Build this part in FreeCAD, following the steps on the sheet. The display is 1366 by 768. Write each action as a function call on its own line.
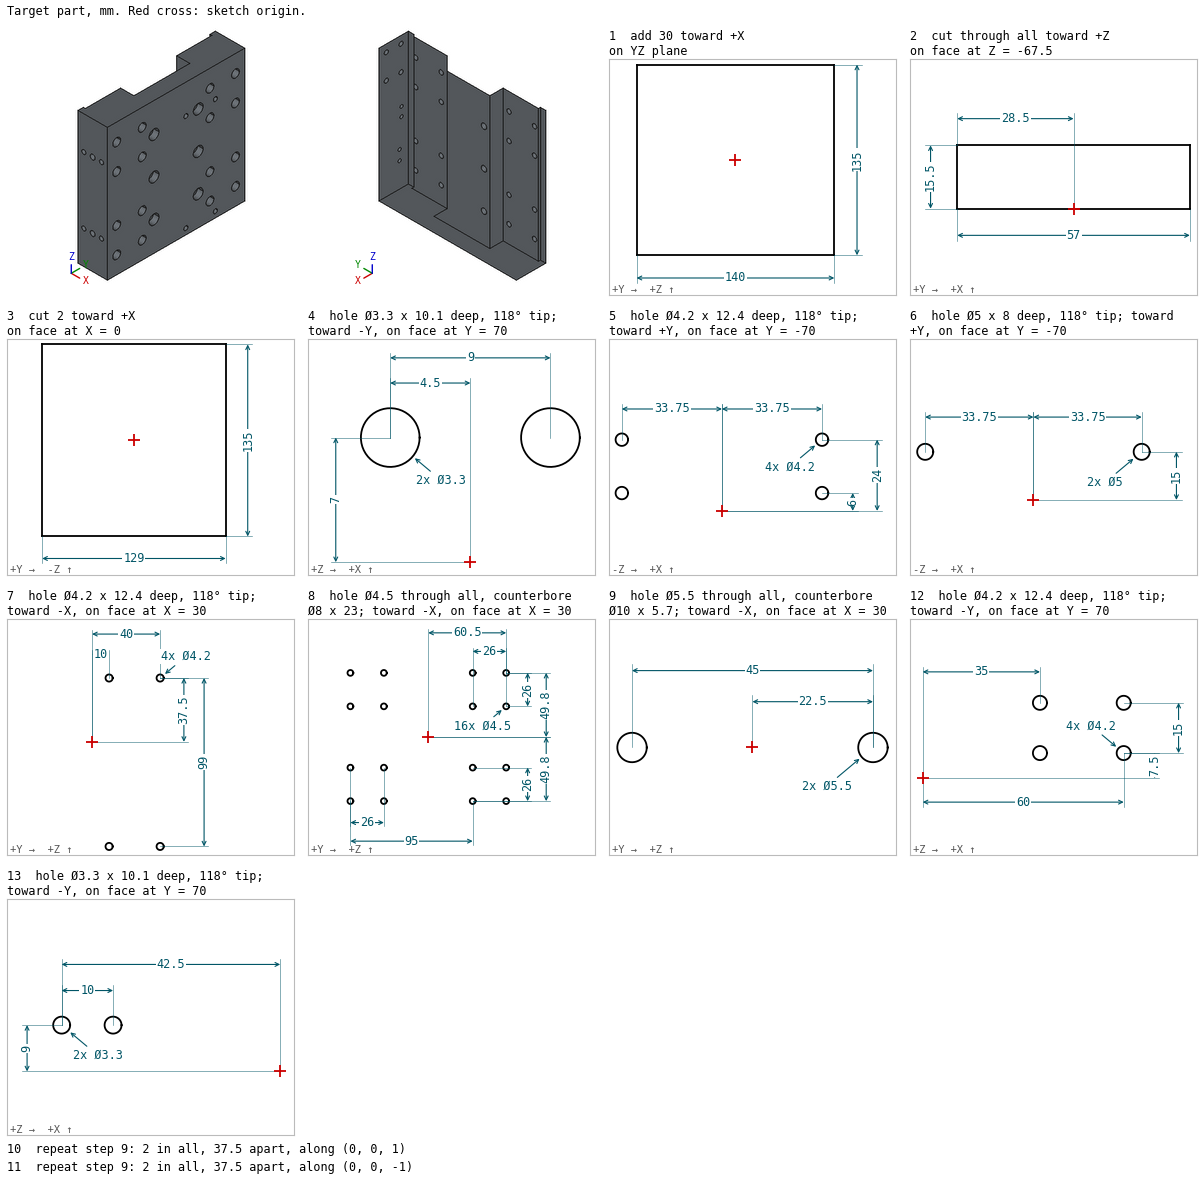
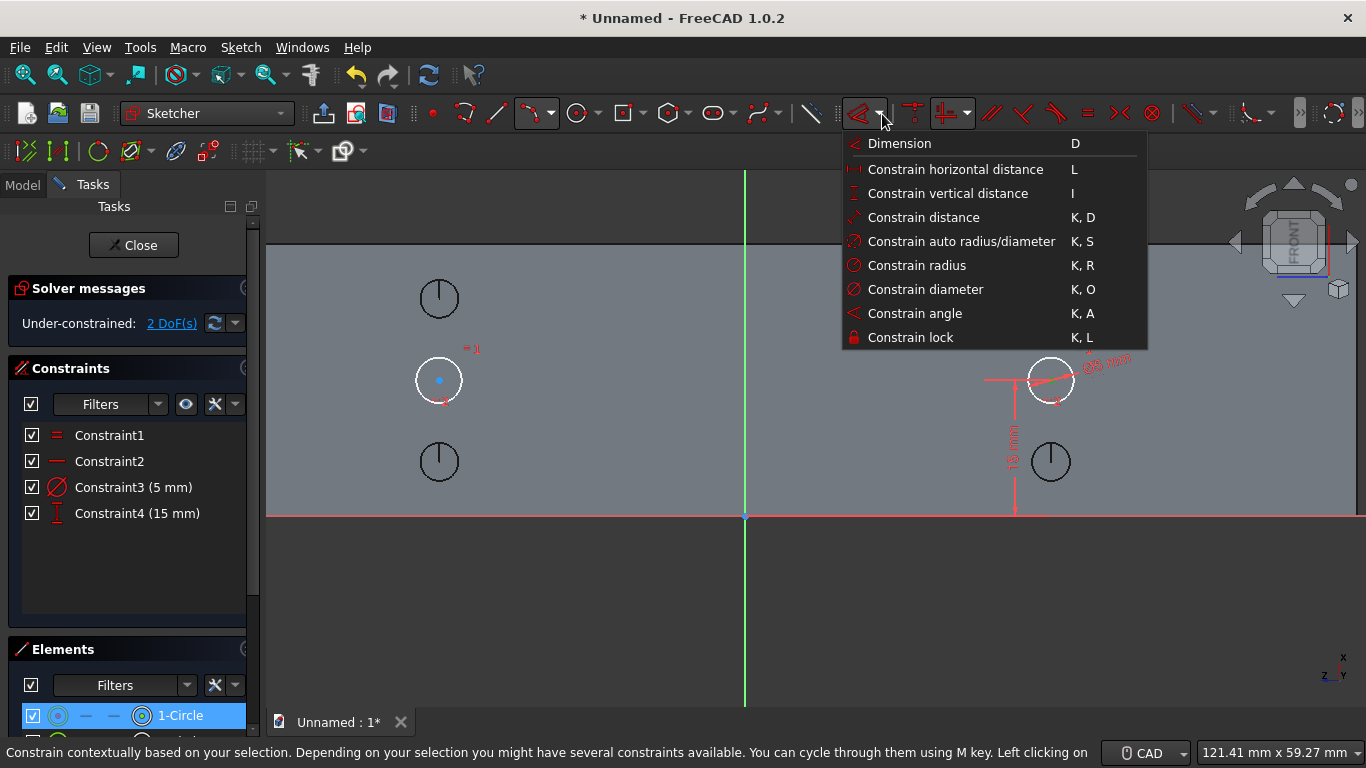
click(995, 169)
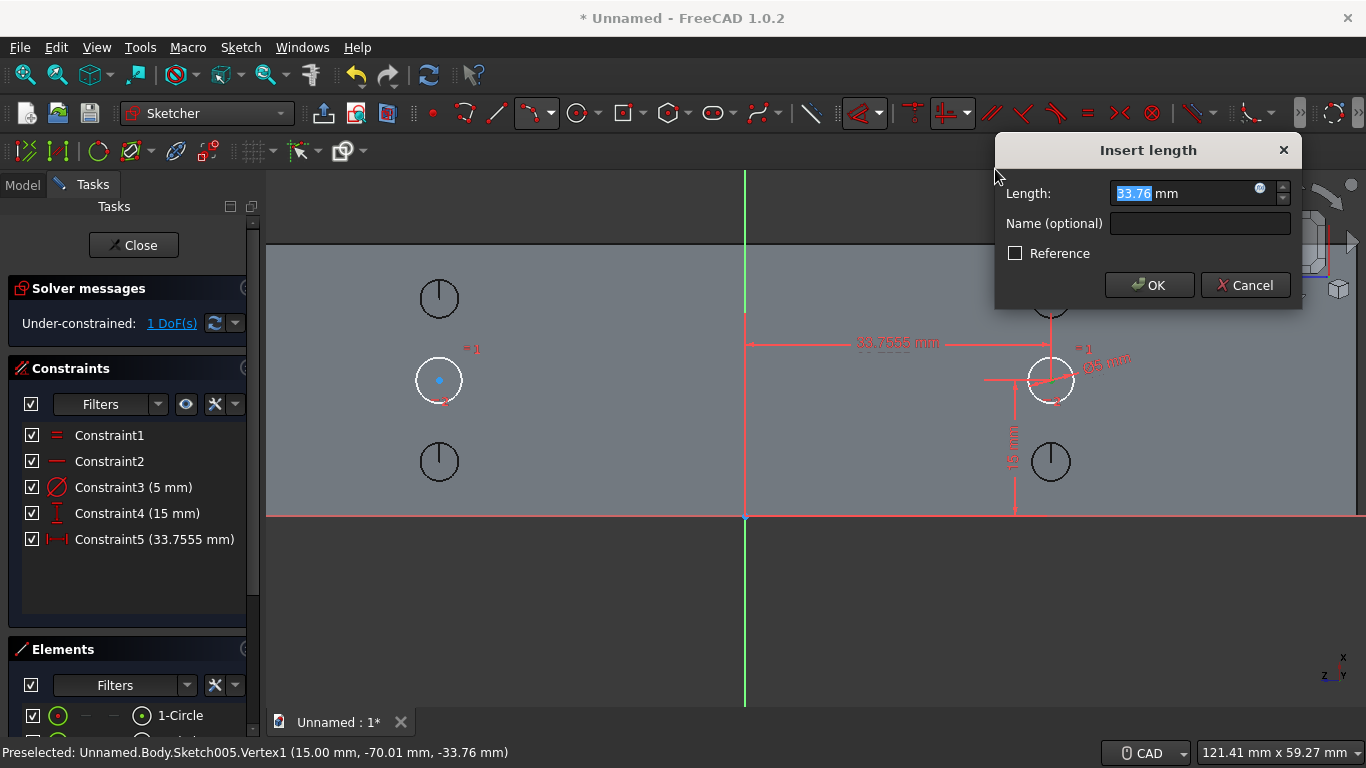
text(33.75)
key(Return)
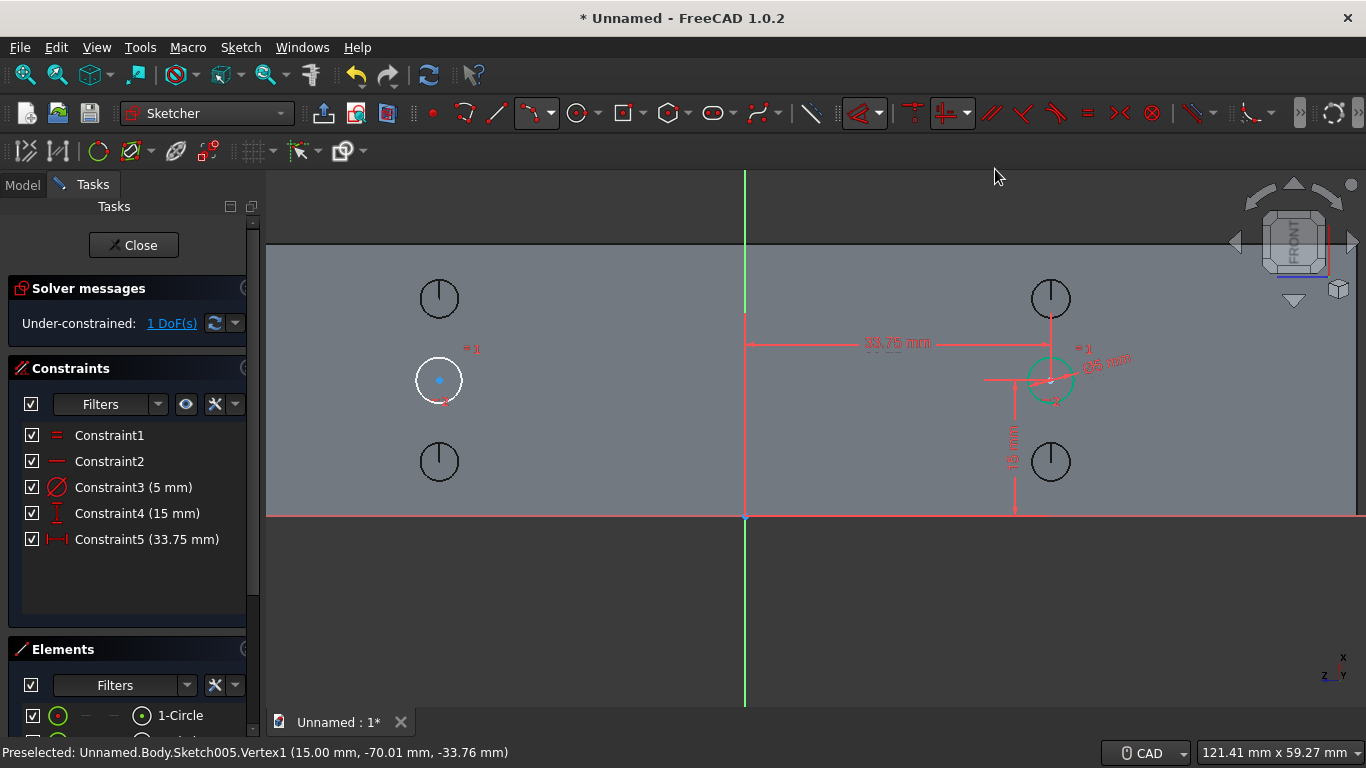
click(439, 380)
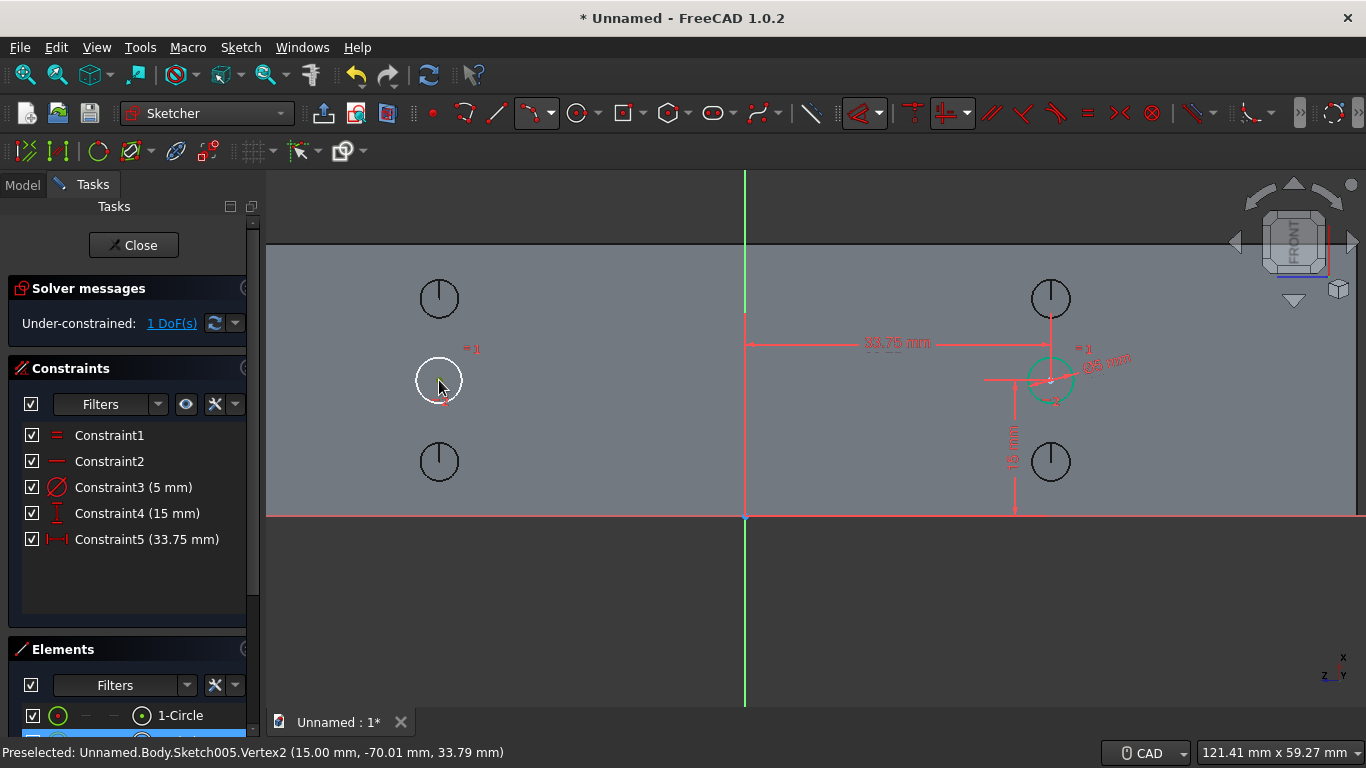
key(l)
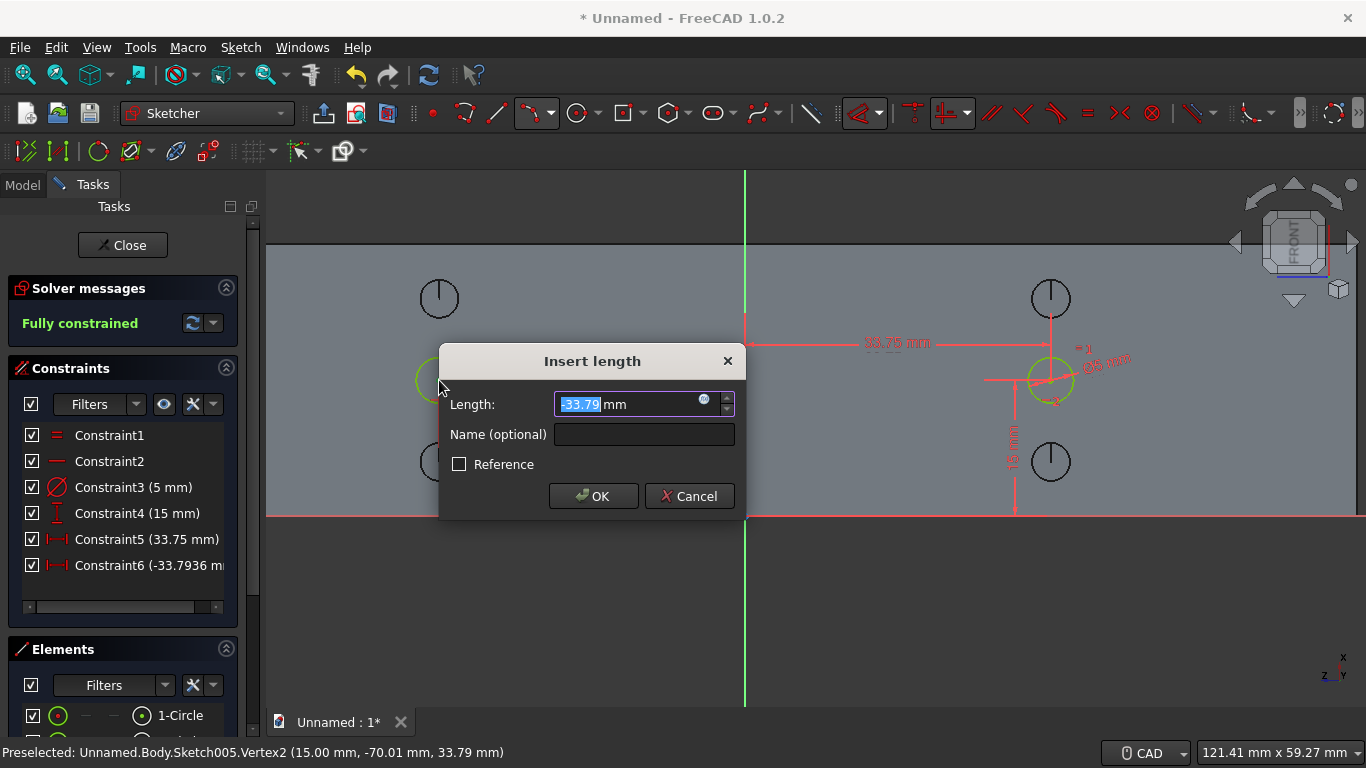
text(-33.75)
key(Return)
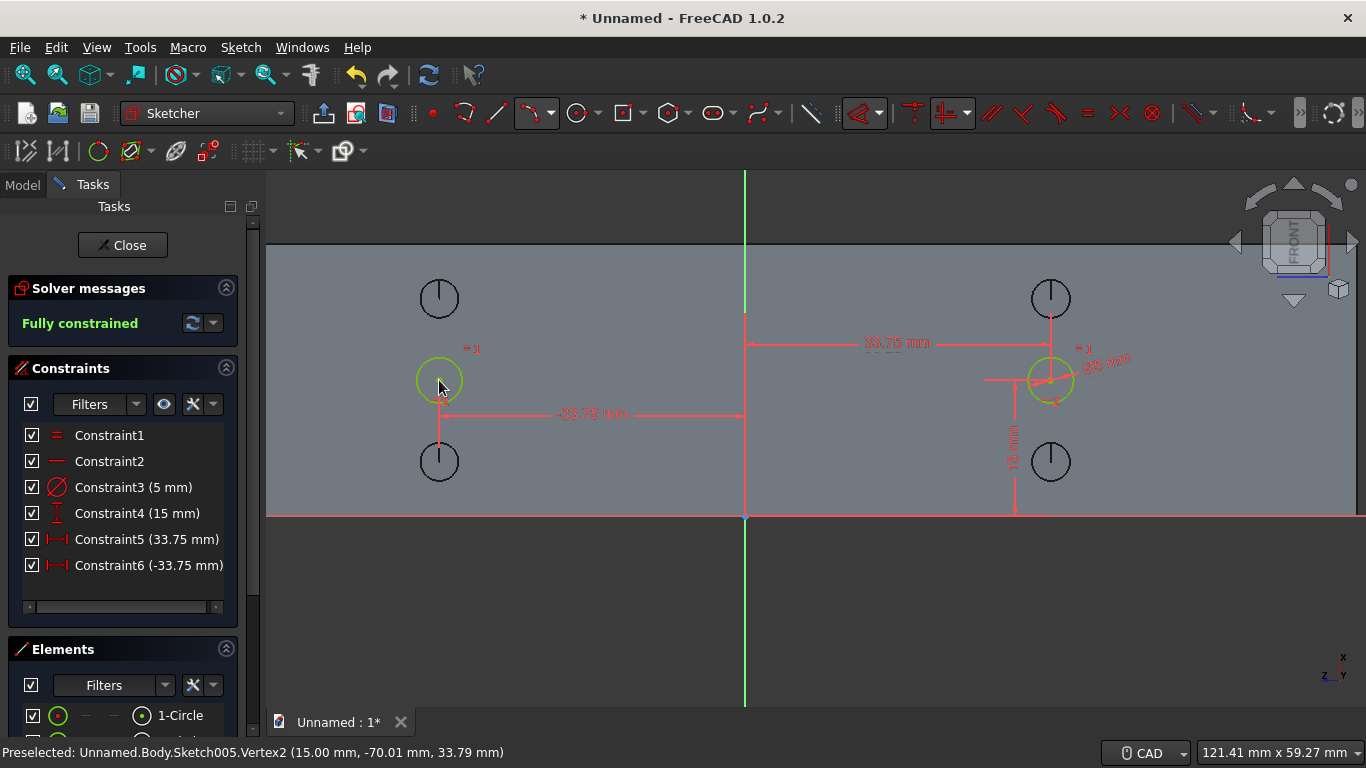
click(123, 245)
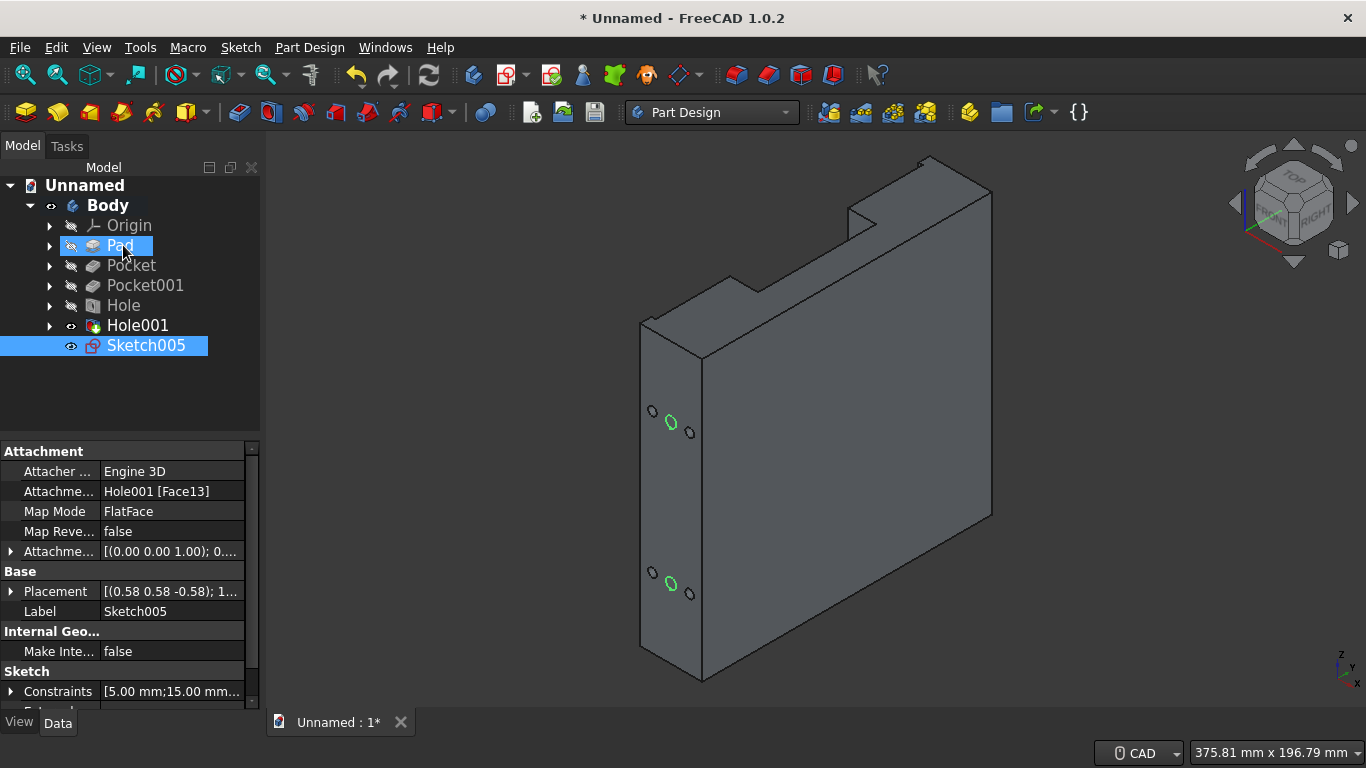
click(272, 112)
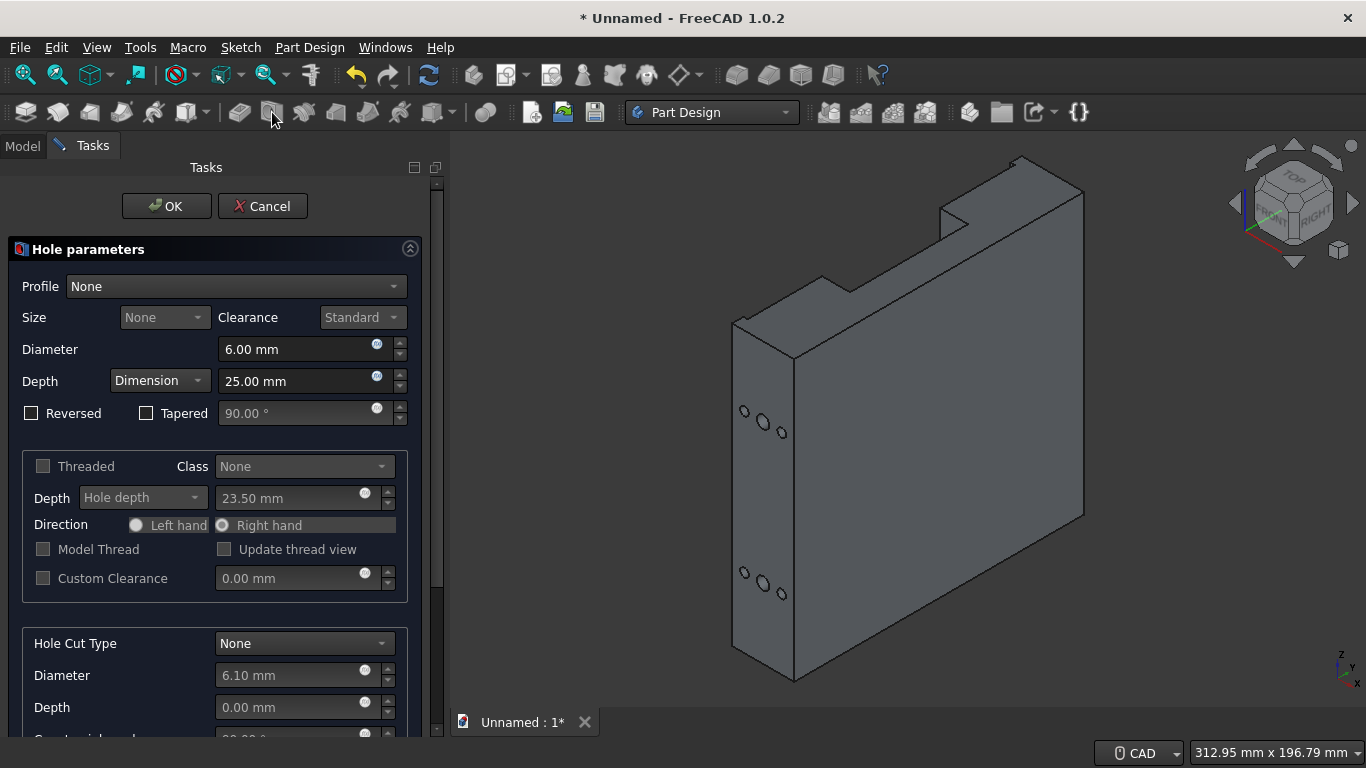
triple_click(305, 349)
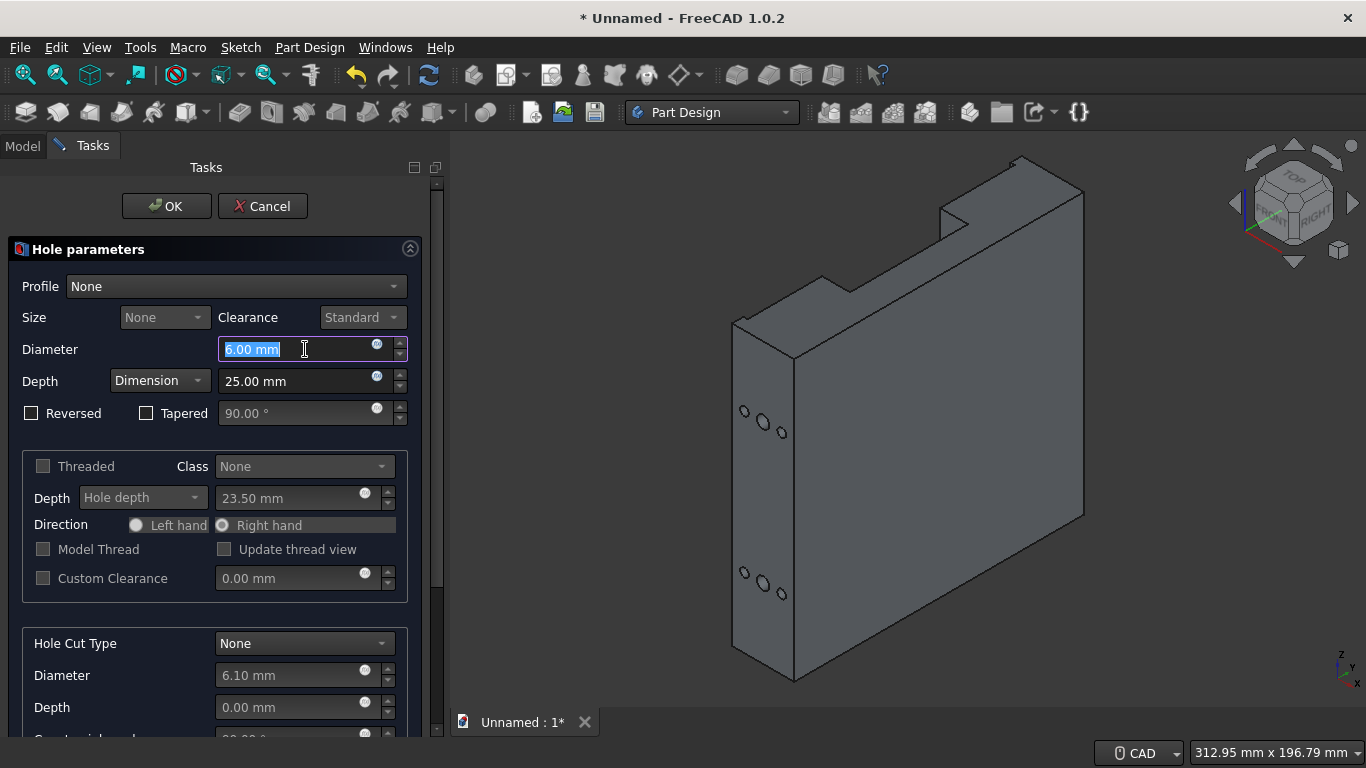
text(5)
key(Tab)